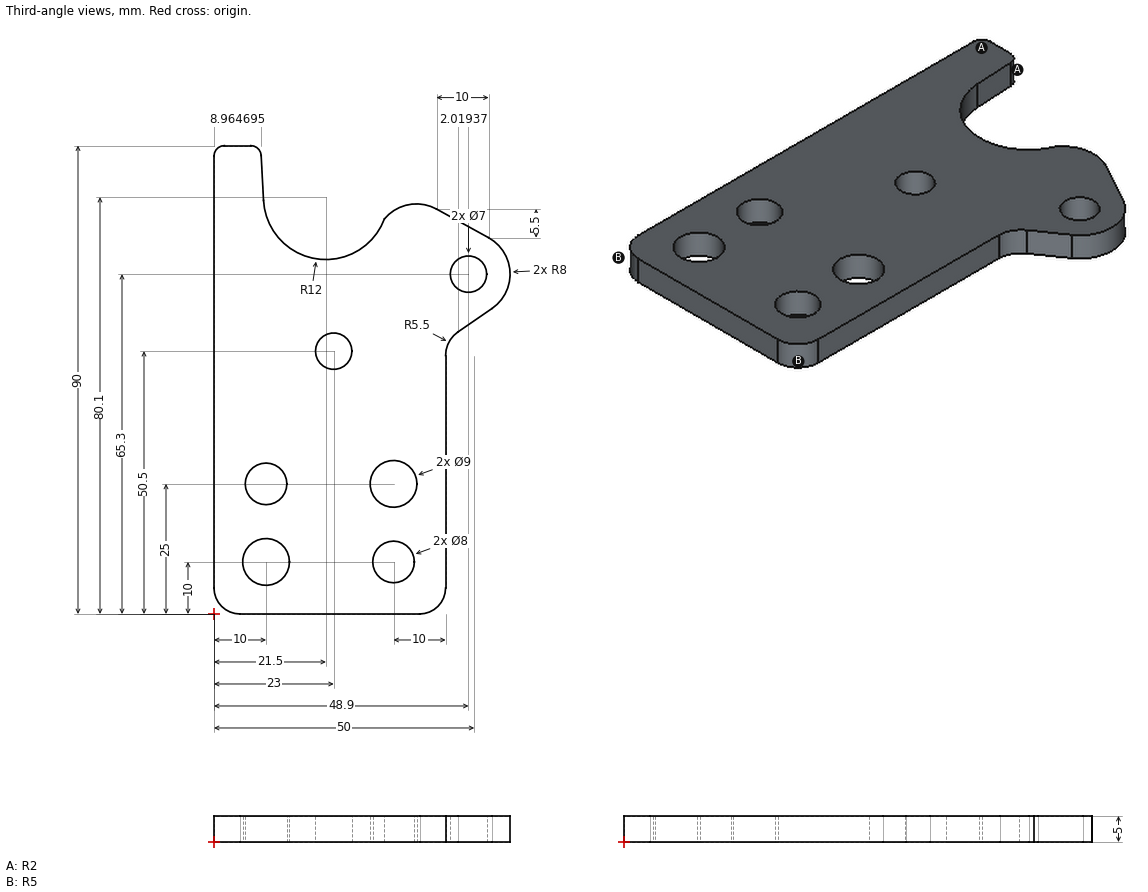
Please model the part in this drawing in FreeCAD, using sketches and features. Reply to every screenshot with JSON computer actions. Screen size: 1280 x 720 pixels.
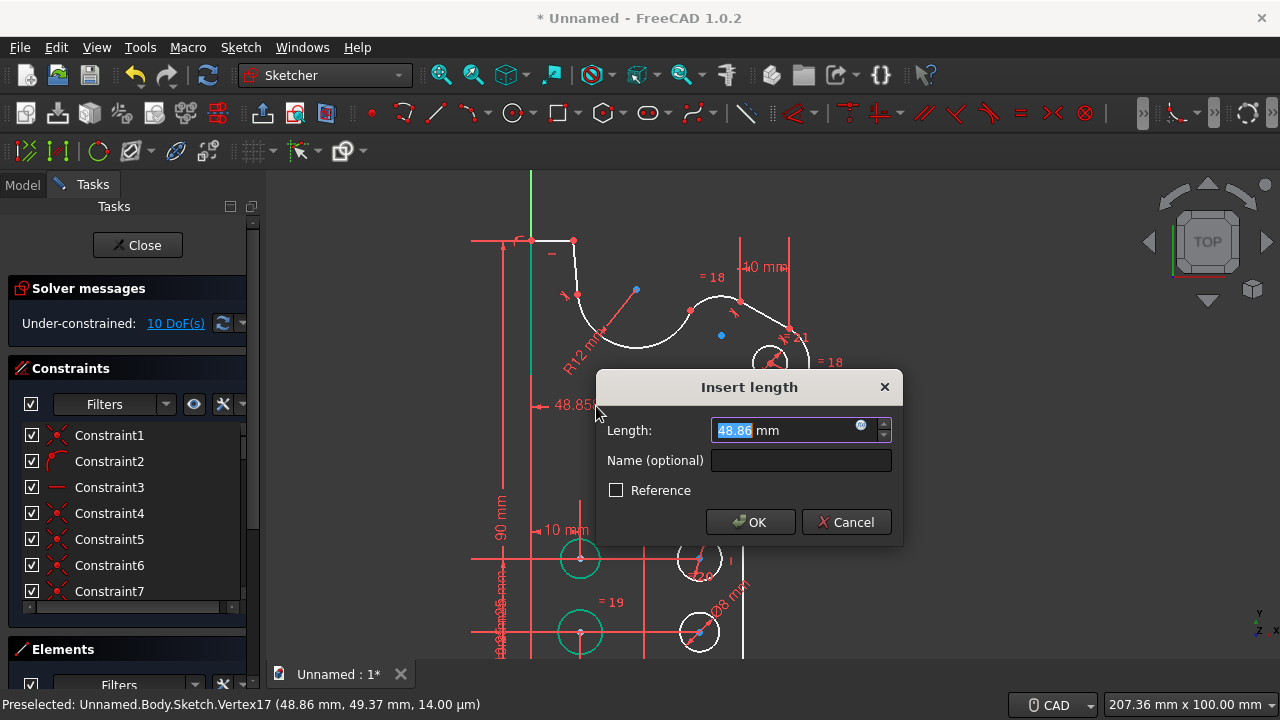
{"action": "type", "text": "50"}
{"action": "key", "text": "Return"}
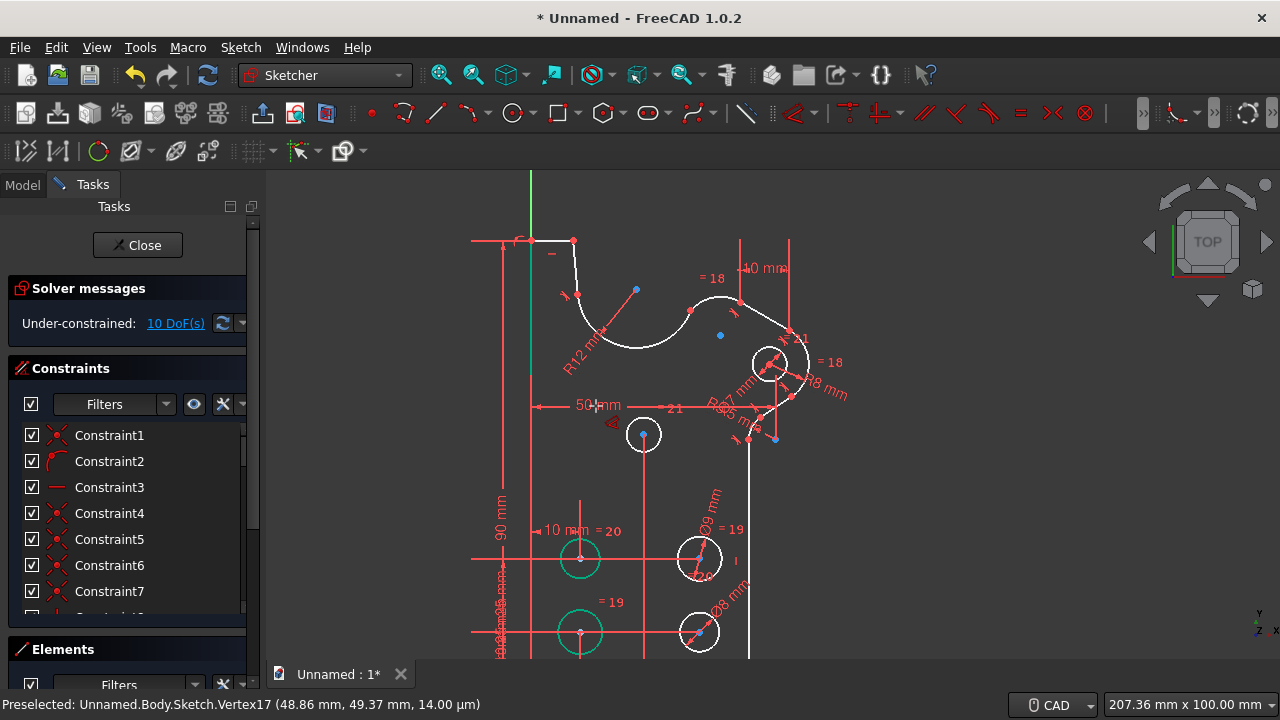
{"action": "scroll", "coordinate": [774, 320], "scroll_direction": "down", "scroll_amount": 2}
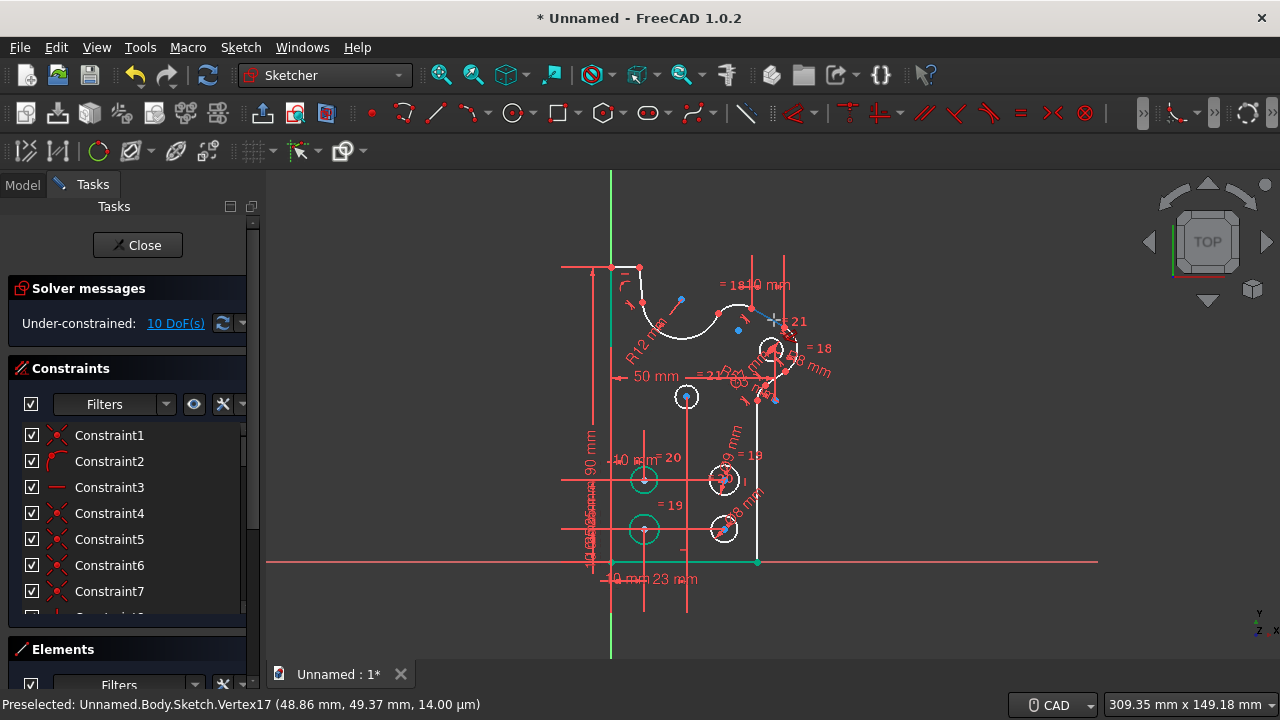
{"action": "left_click", "coordinate": [757, 562]}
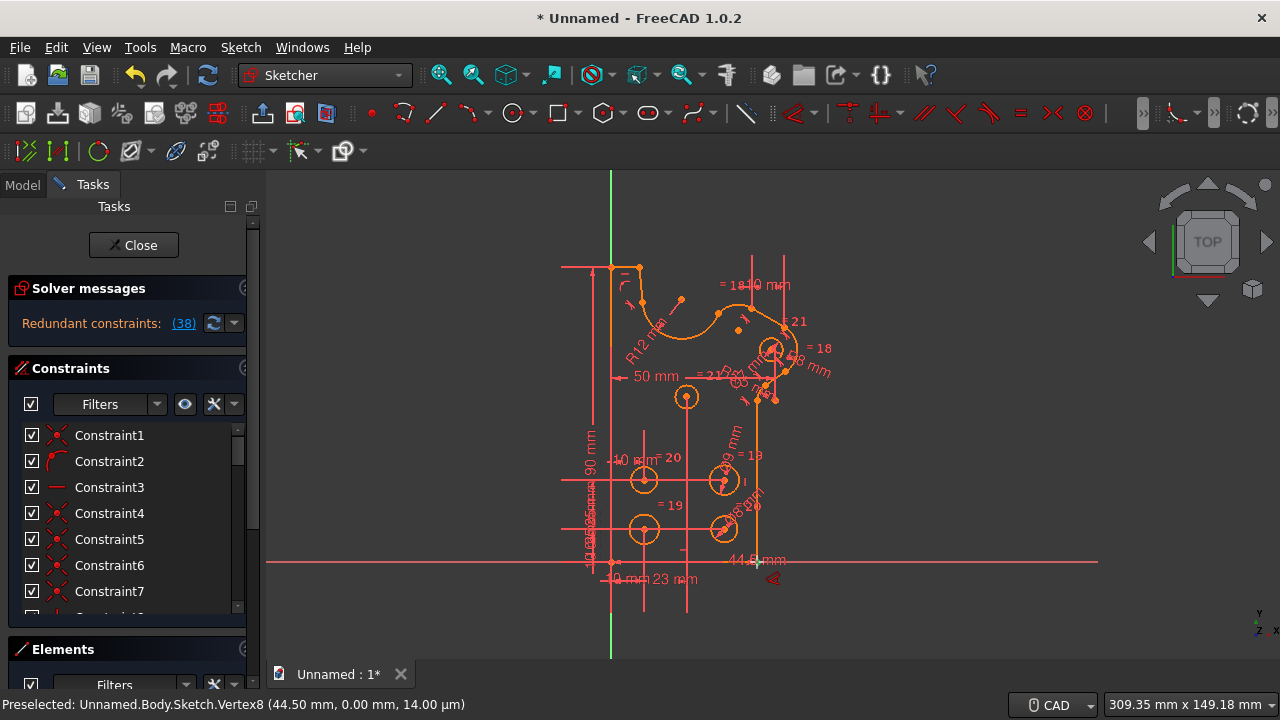
{"action": "left_click", "coordinate": [724, 529]}
{"action": "left_click", "coordinate": [748, 596]}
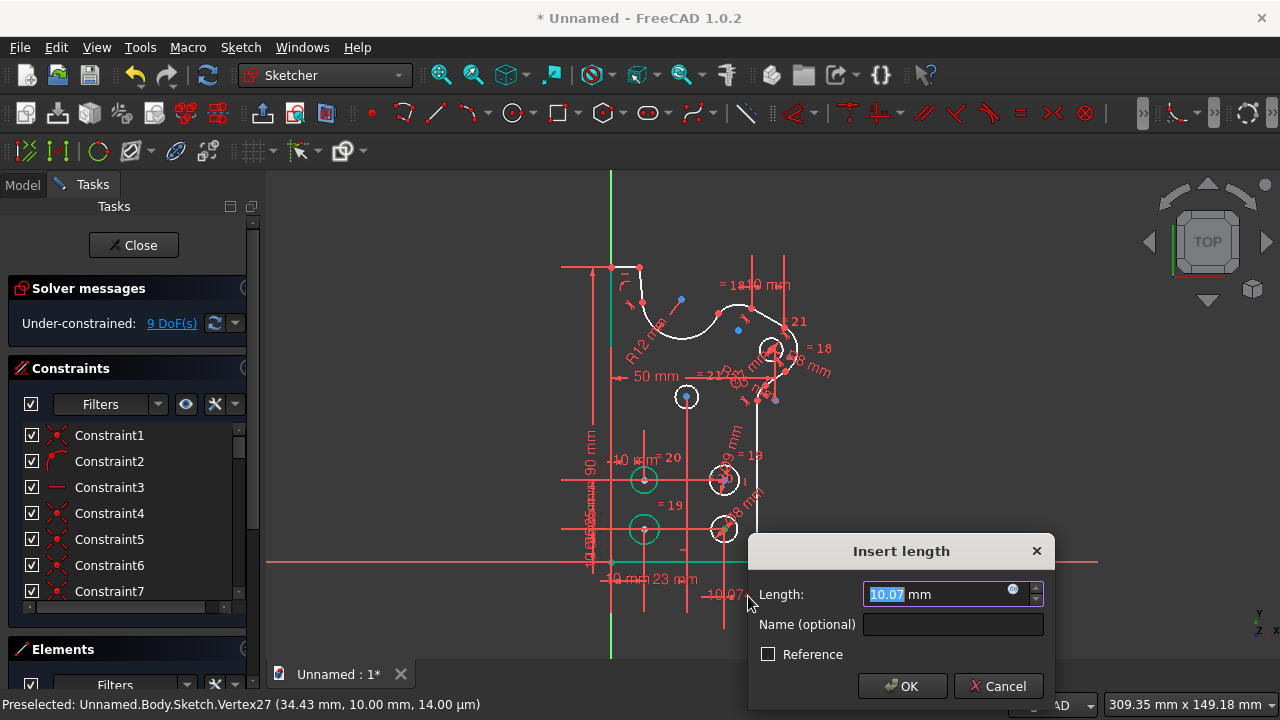
{"action": "type", "text": "10"}
{"action": "key", "text": "Return"}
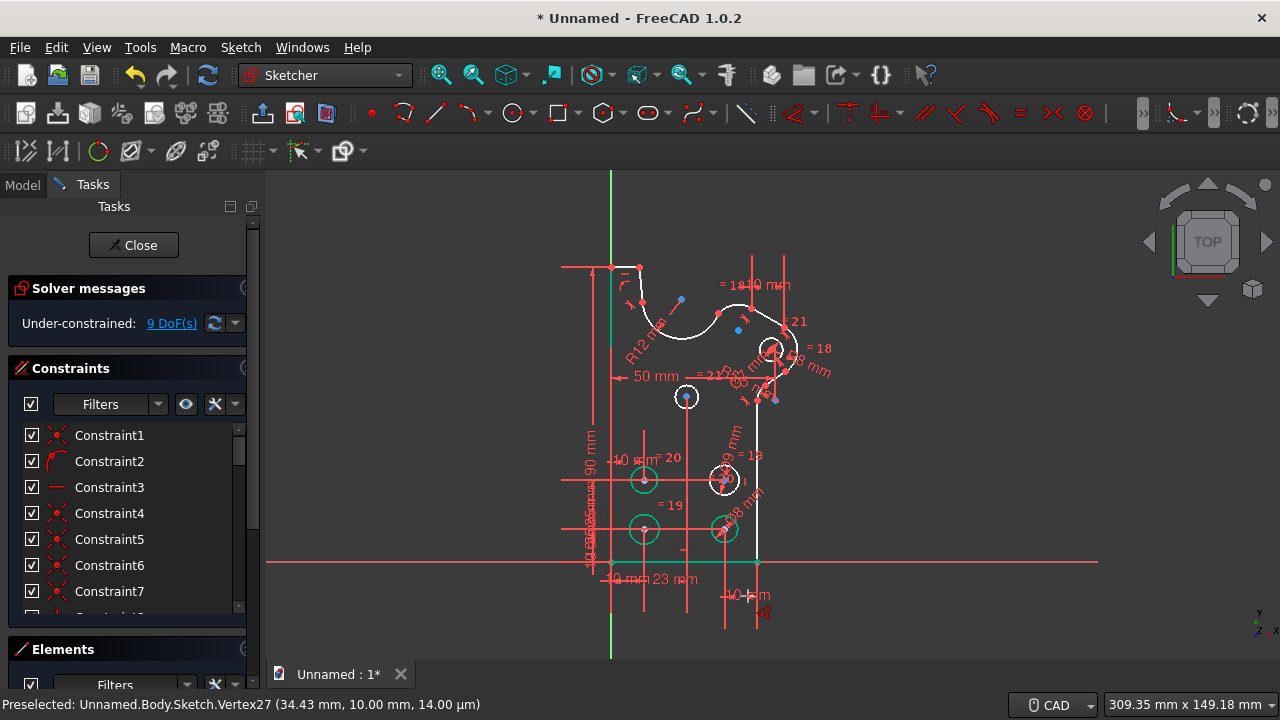
{"action": "left_click", "coordinate": [757, 400]}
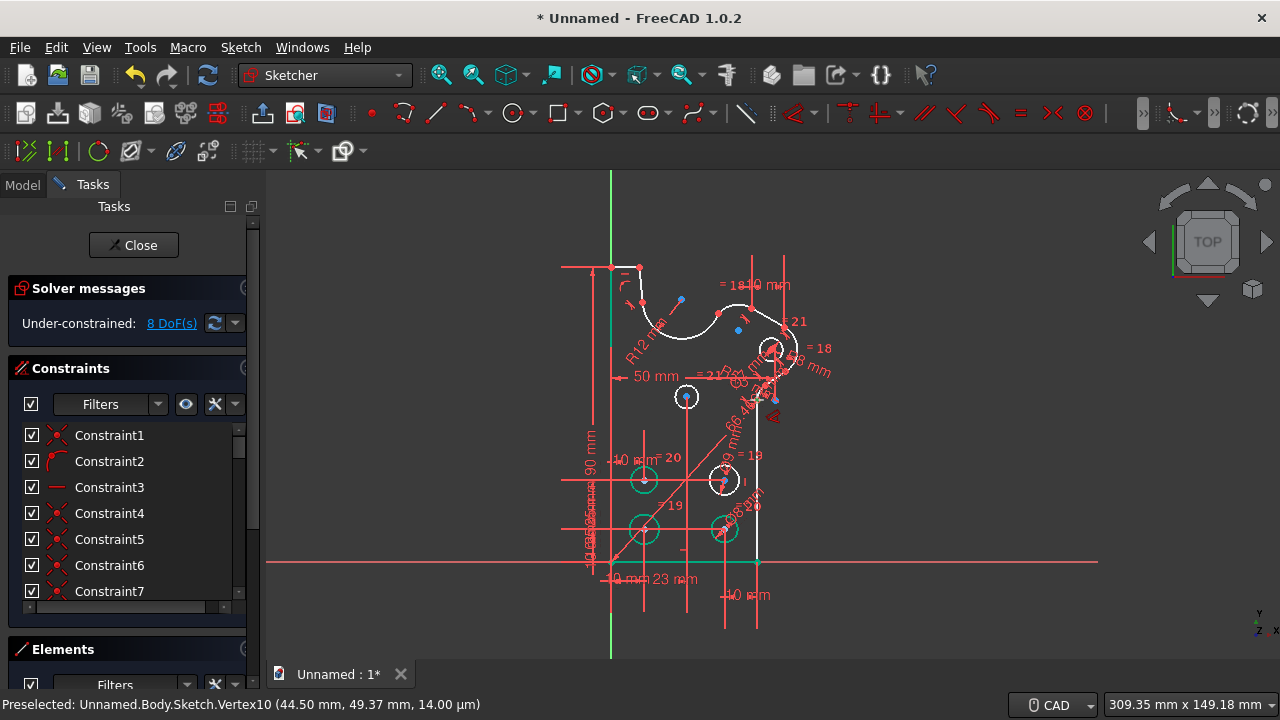
{"action": "left_click", "coordinate": [724, 480]}
{"action": "left_click", "coordinate": [741, 342]}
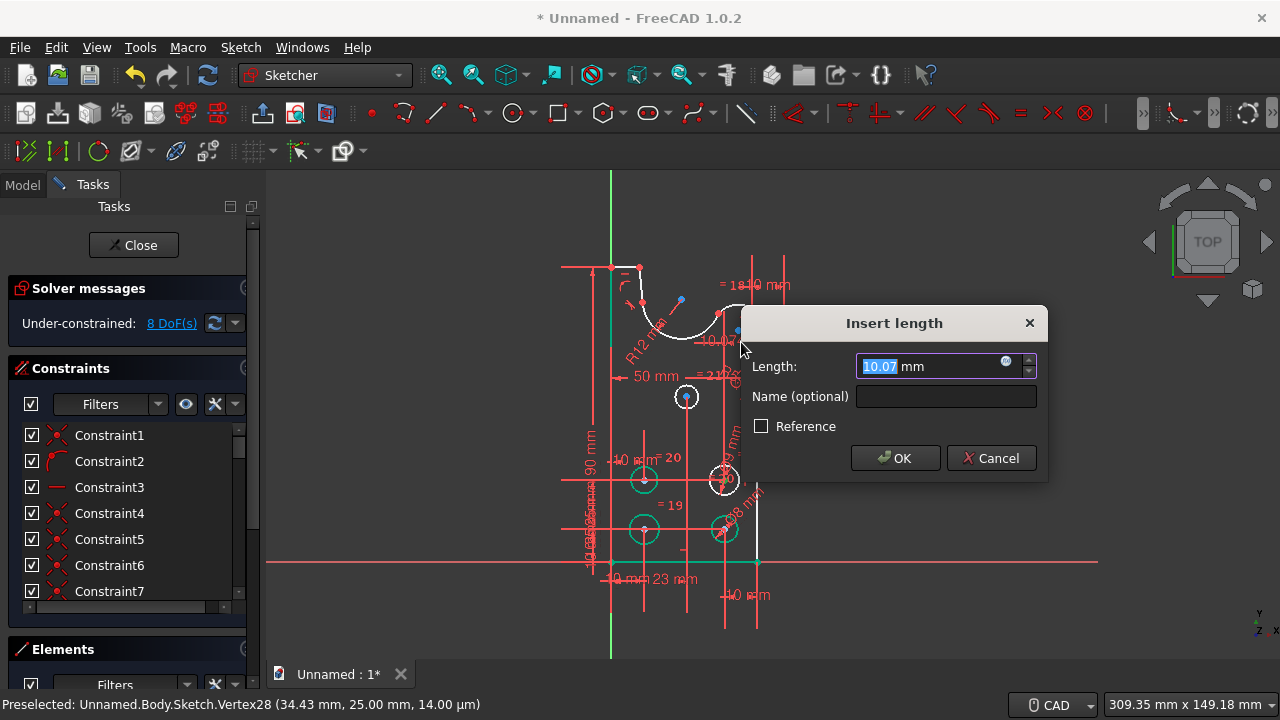
{"action": "type", "text": "10"}
{"action": "key", "text": "Return"}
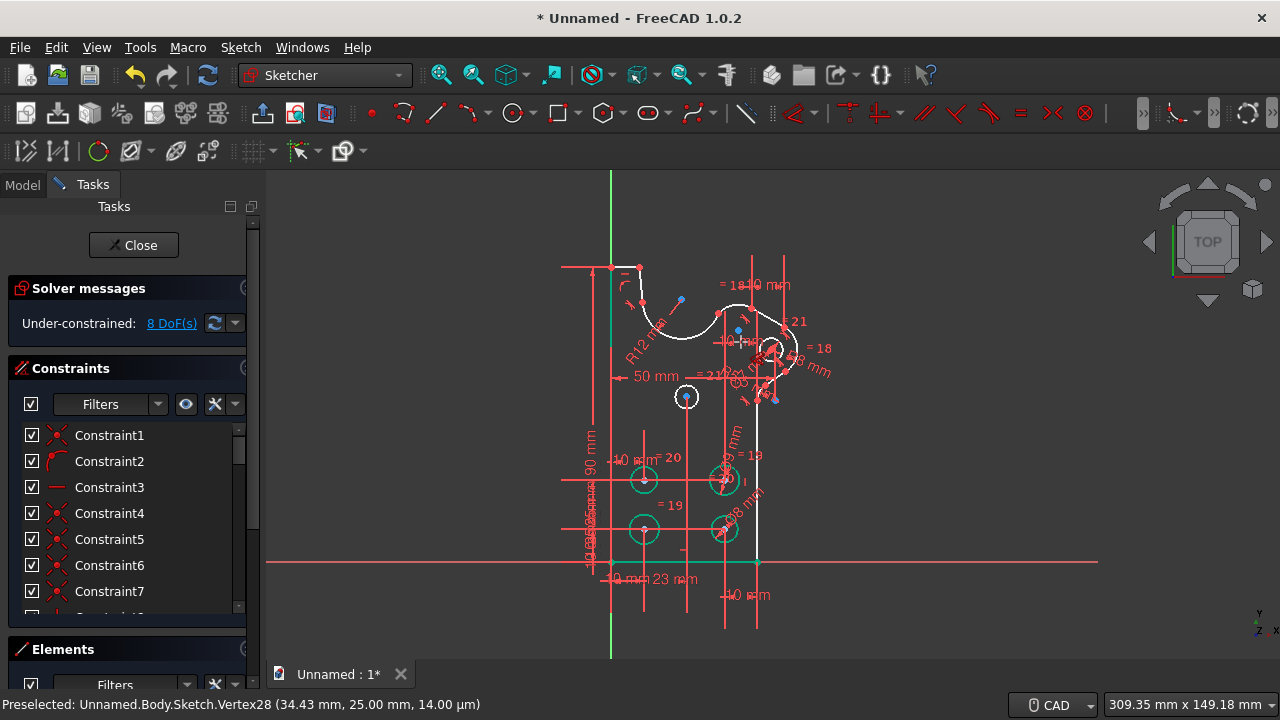
{"action": "scroll", "coordinate": [775, 321], "scroll_direction": "up", "scroll_amount": 4}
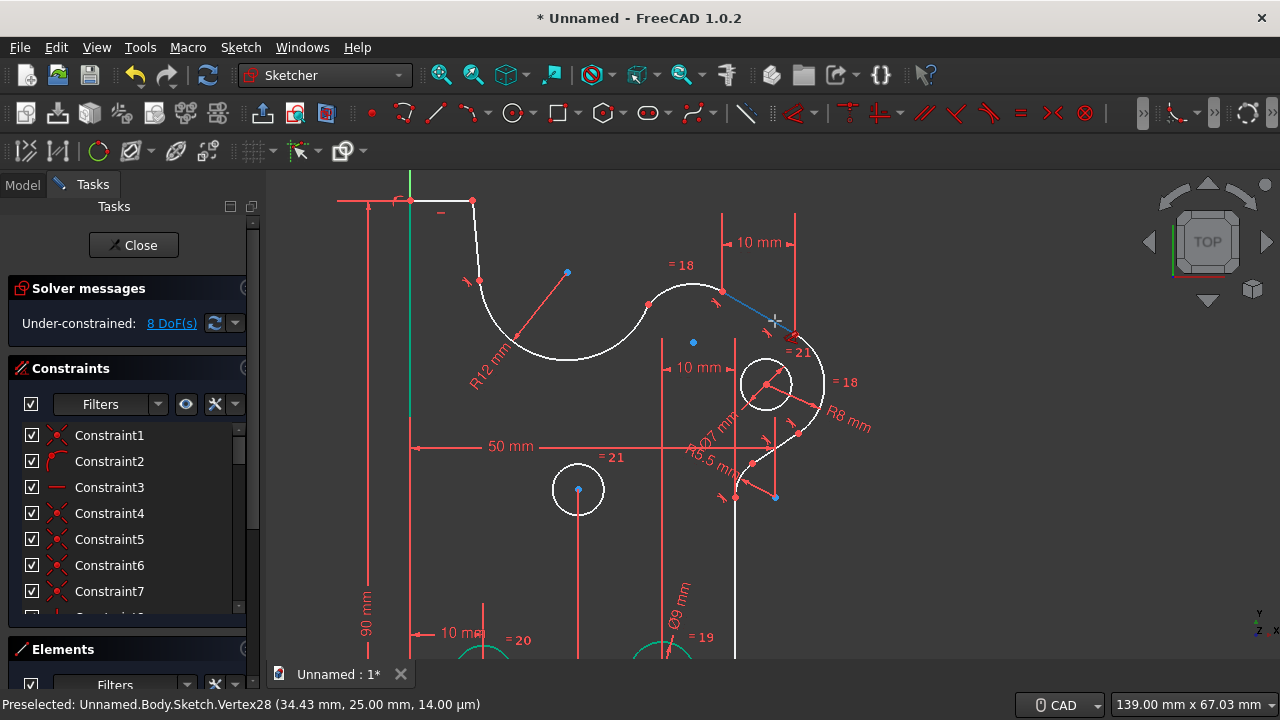
{"action": "left_click", "coordinate": [773, 321]}
{"action": "left_click", "coordinate": [829, 313]}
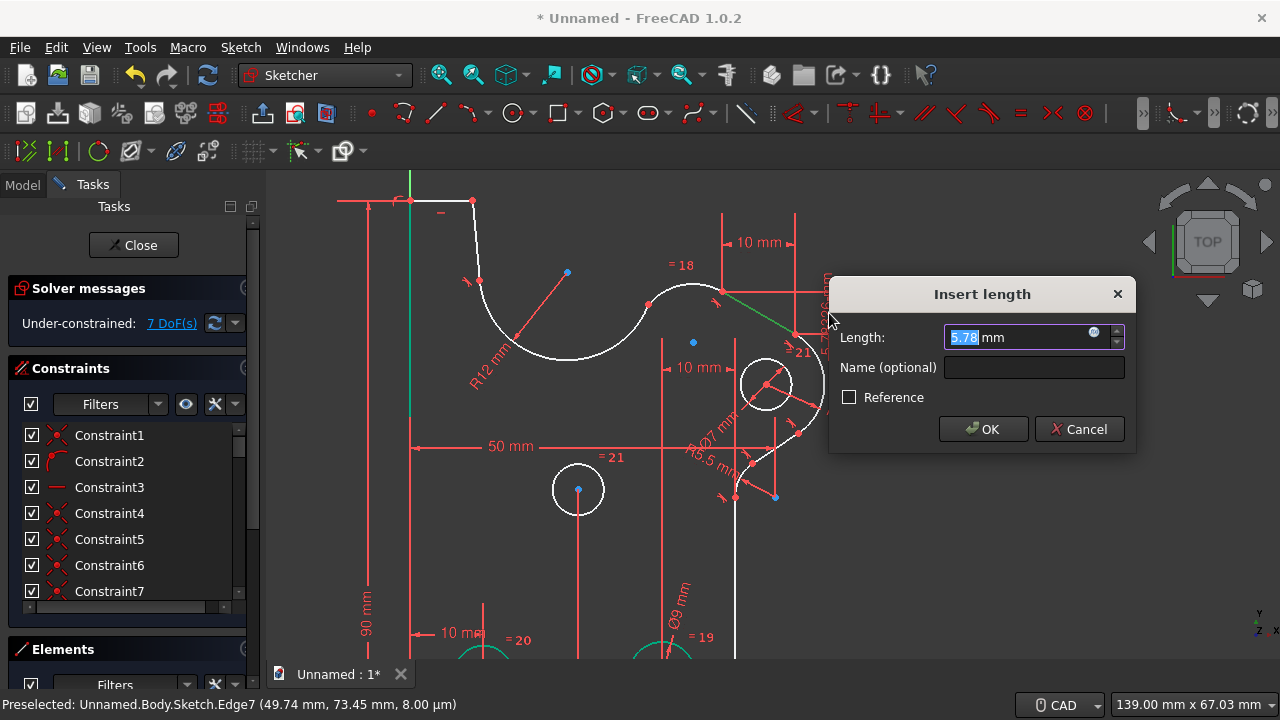
{"action": "type", "text": "5.5"}
{"action": "key", "text": "Return"}